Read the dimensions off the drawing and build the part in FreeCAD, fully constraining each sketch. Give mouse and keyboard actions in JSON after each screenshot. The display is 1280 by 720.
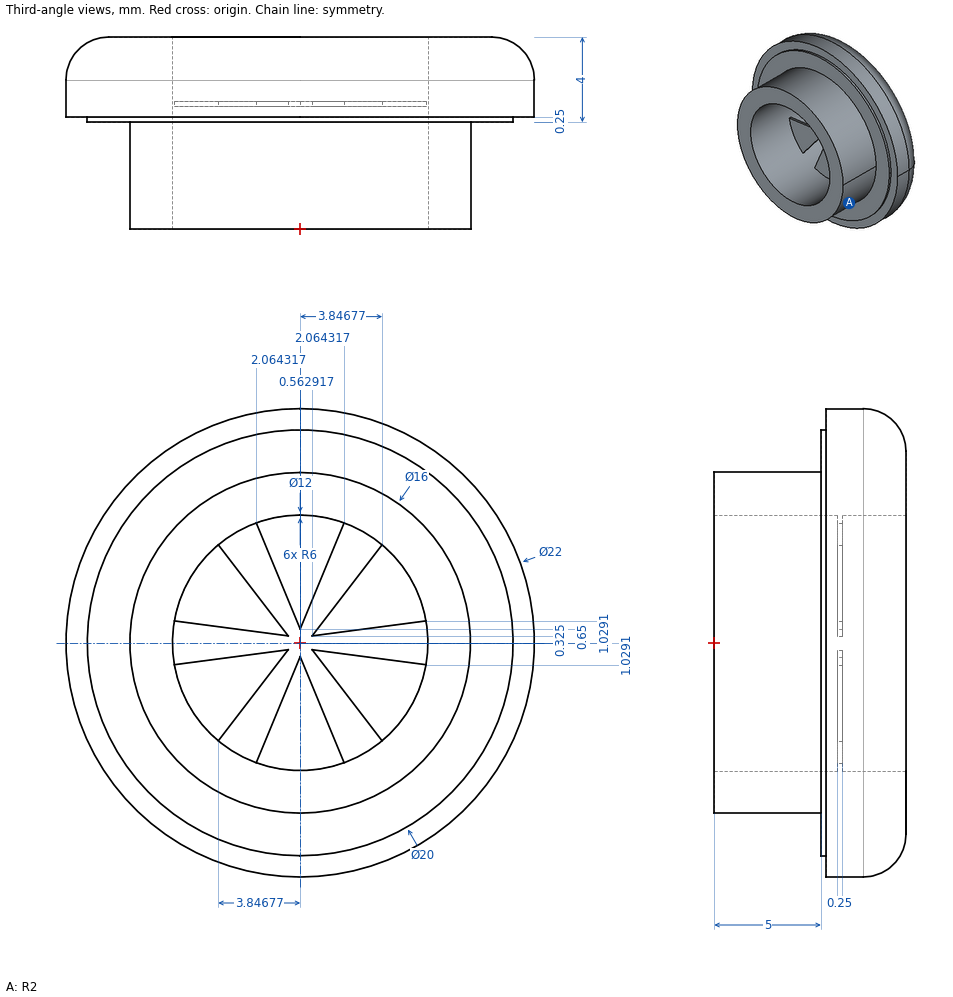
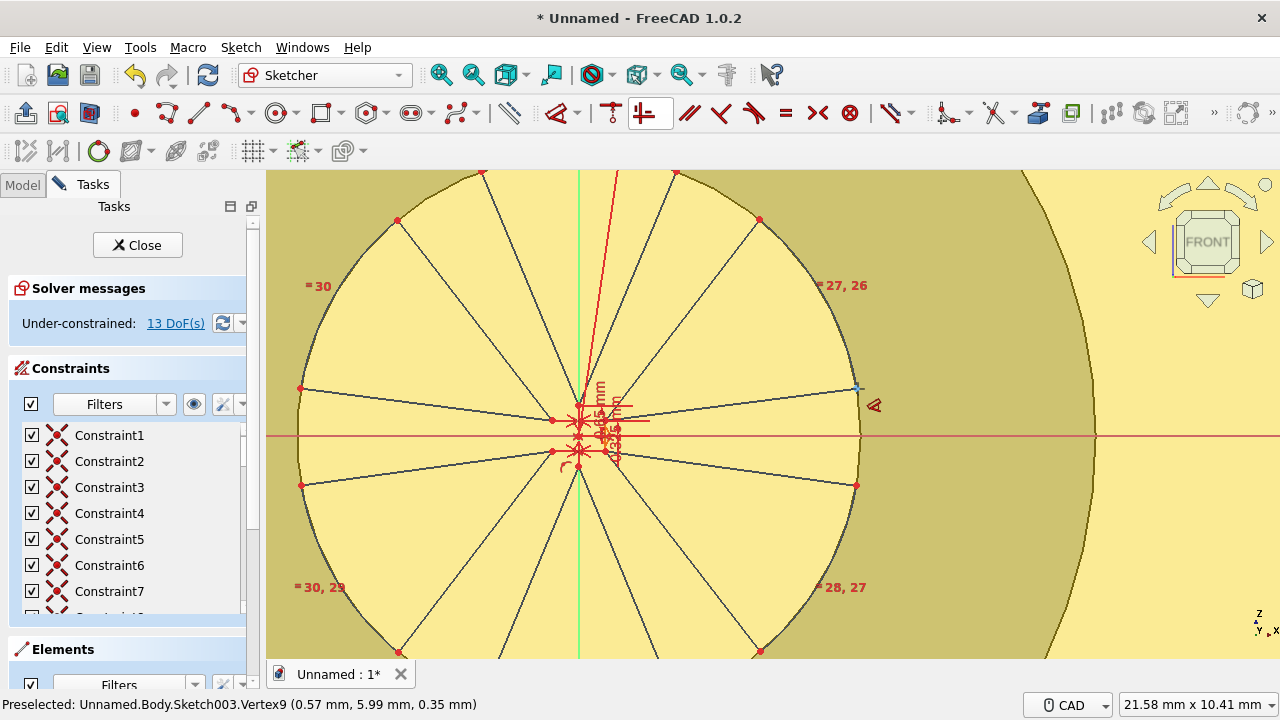
{"action": "left_click", "coordinate": [857, 389]}
{"action": "left_click", "coordinate": [891, 412]}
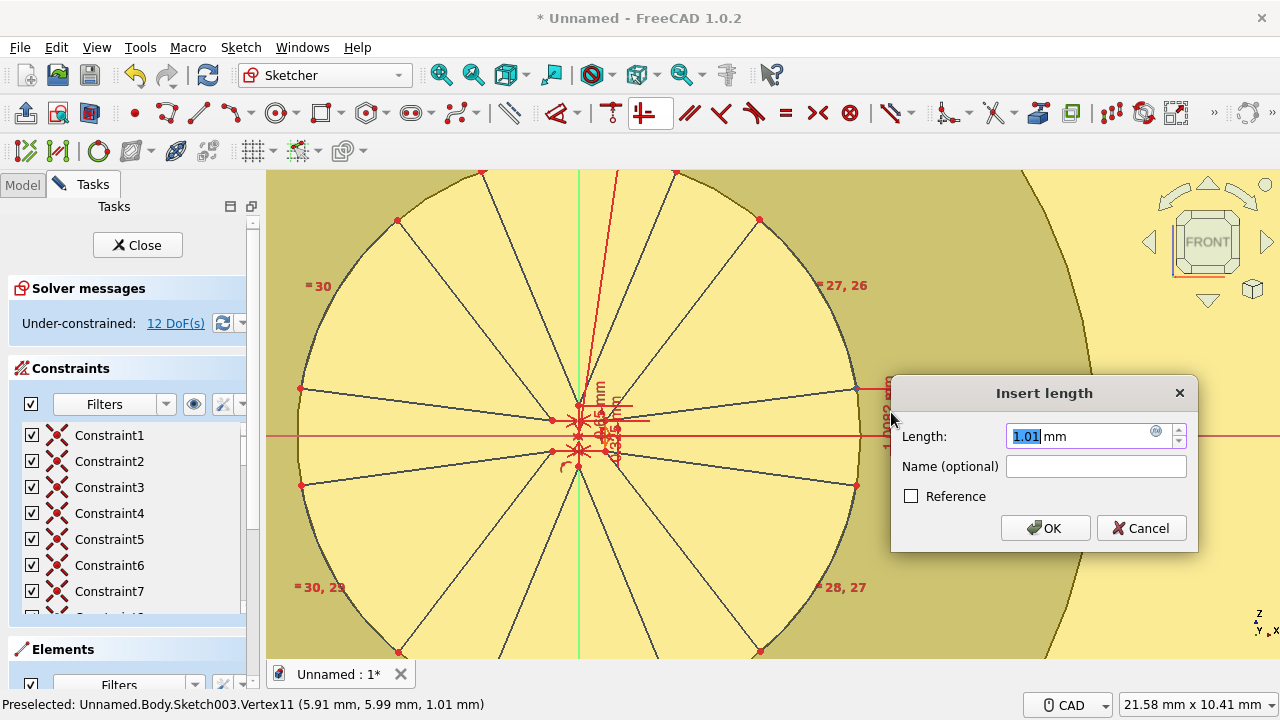
{"action": "type", "text": "1.0291"}
{"action": "key", "text": "Return"}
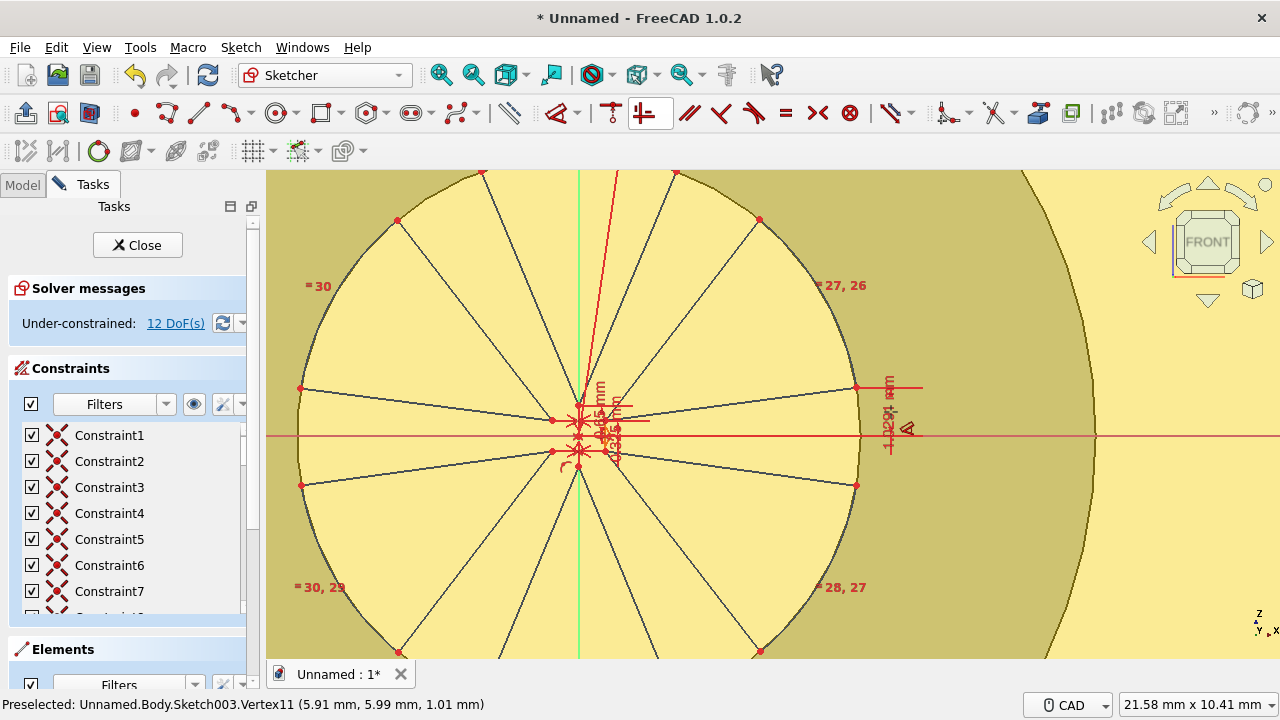
{"action": "left_click", "coordinate": [856, 486]}
{"action": "left_click", "coordinate": [890, 461]}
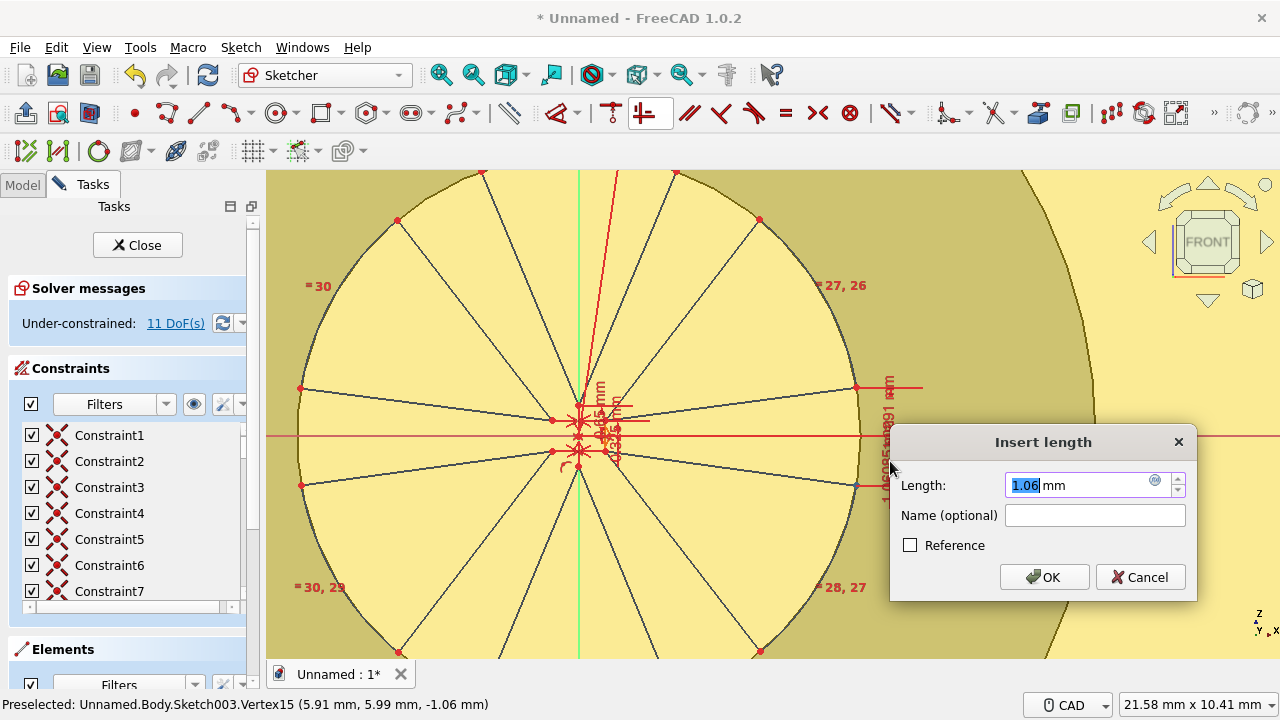
{"action": "type", "text": "1.0291"}
{"action": "key", "text": "Return"}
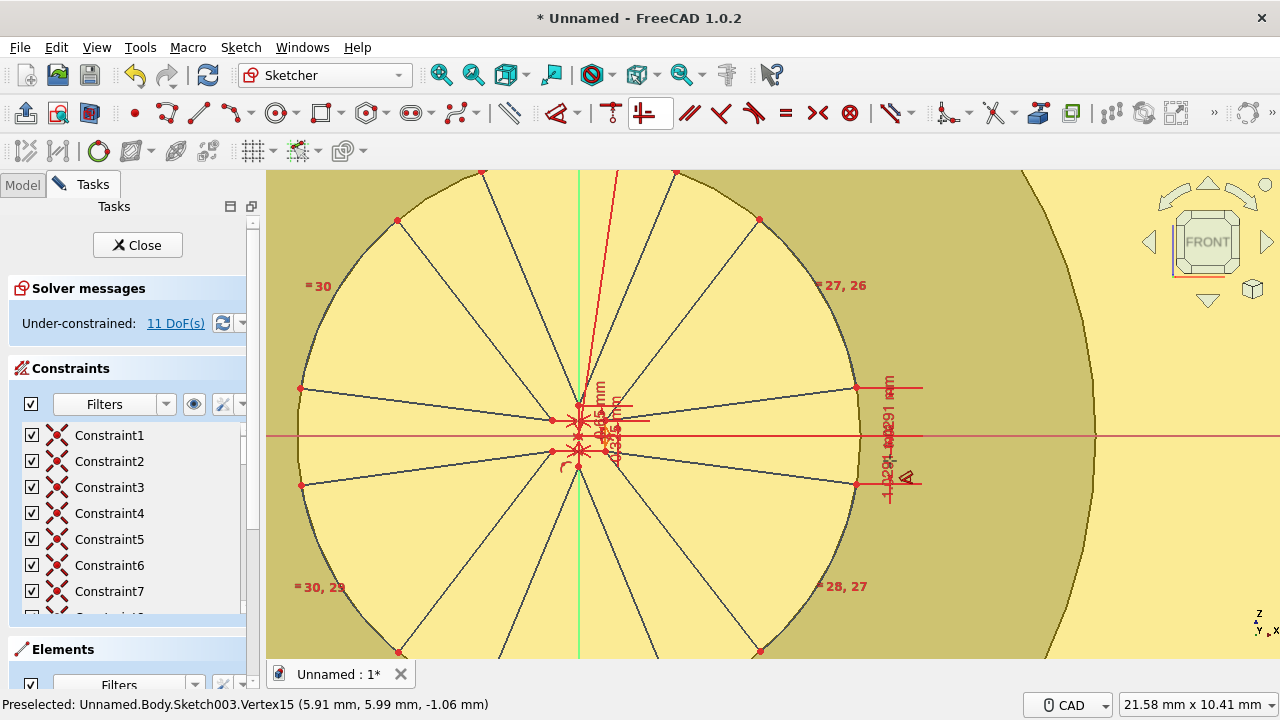
{"action": "left_click", "coordinate": [301, 486]}
{"action": "left_click", "coordinate": [661, 472]}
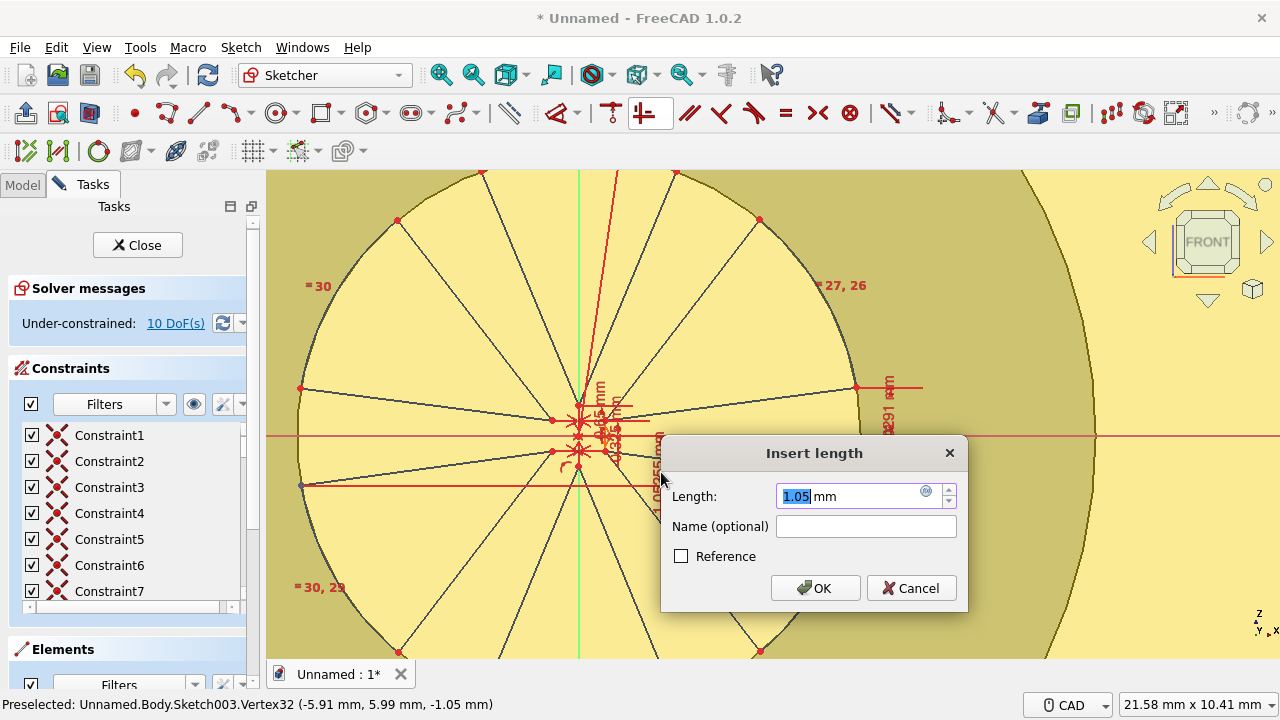
{"action": "type", "text": "1.0291"}
{"action": "key", "text": "Return"}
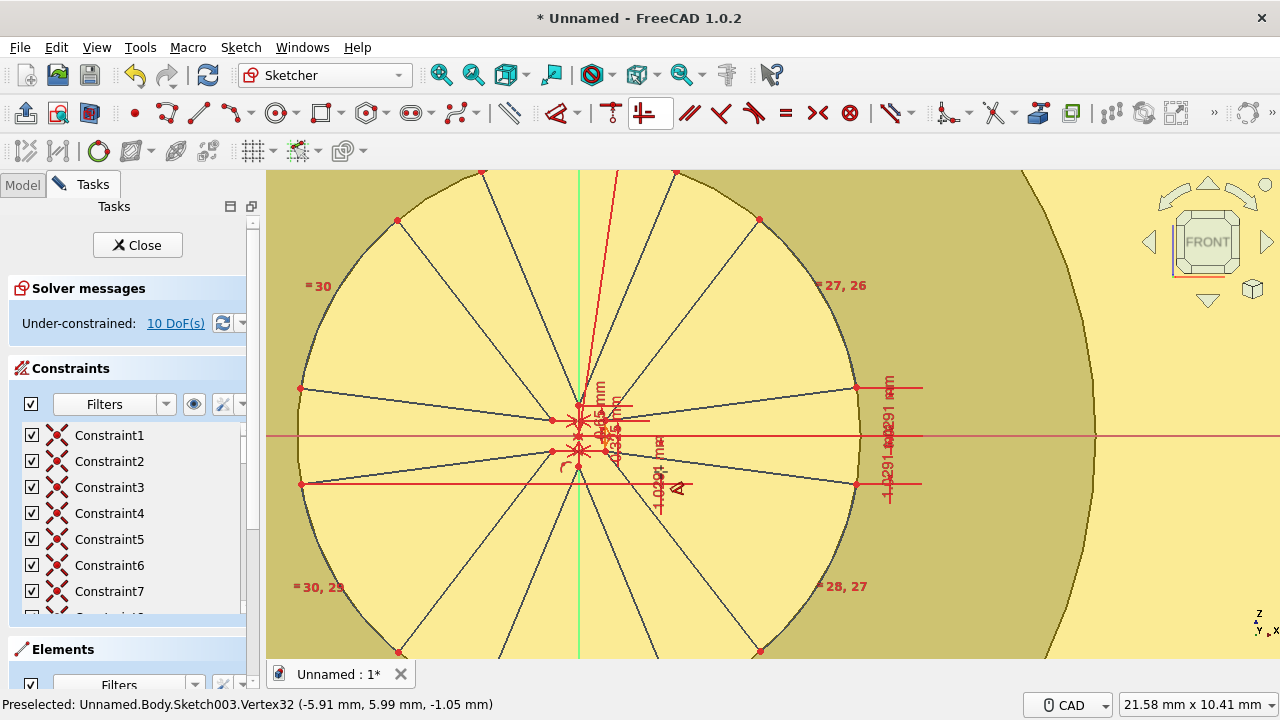
{"action": "left_click", "coordinate": [301, 389]}
{"action": "left_click", "coordinate": [685, 396]}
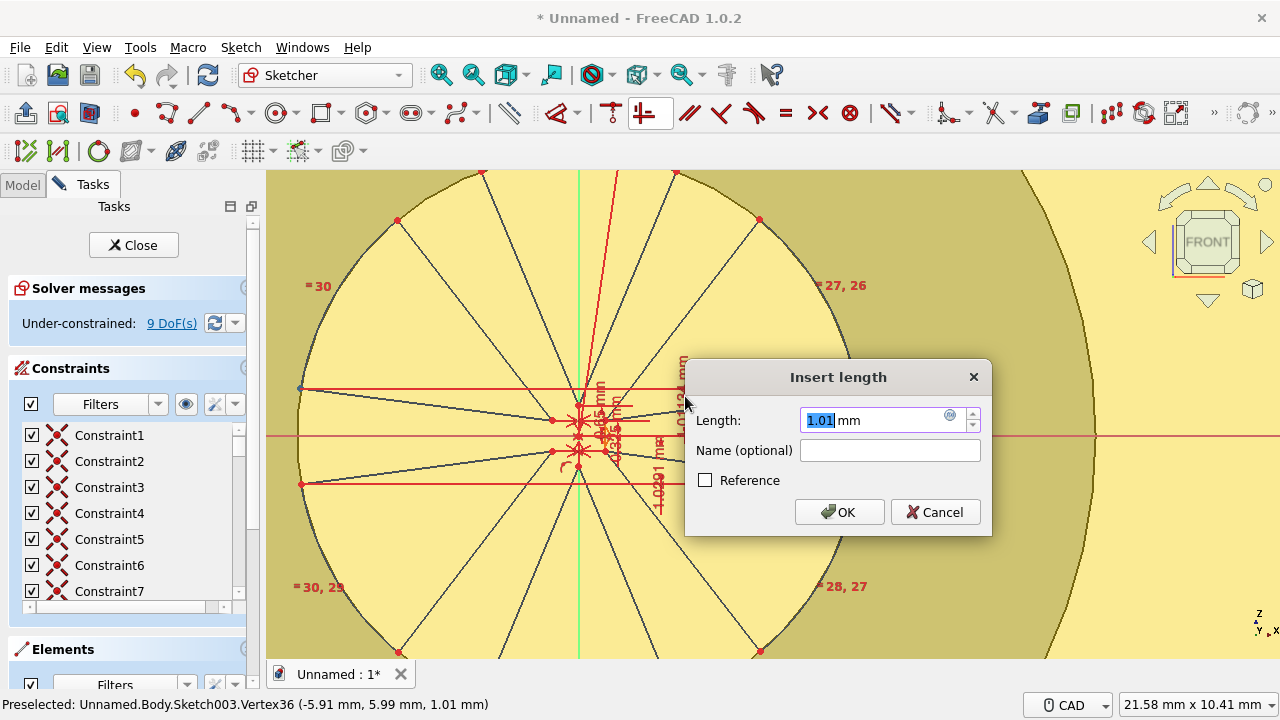
{"action": "type", "text": "1.0291"}
{"action": "key", "text": "Return"}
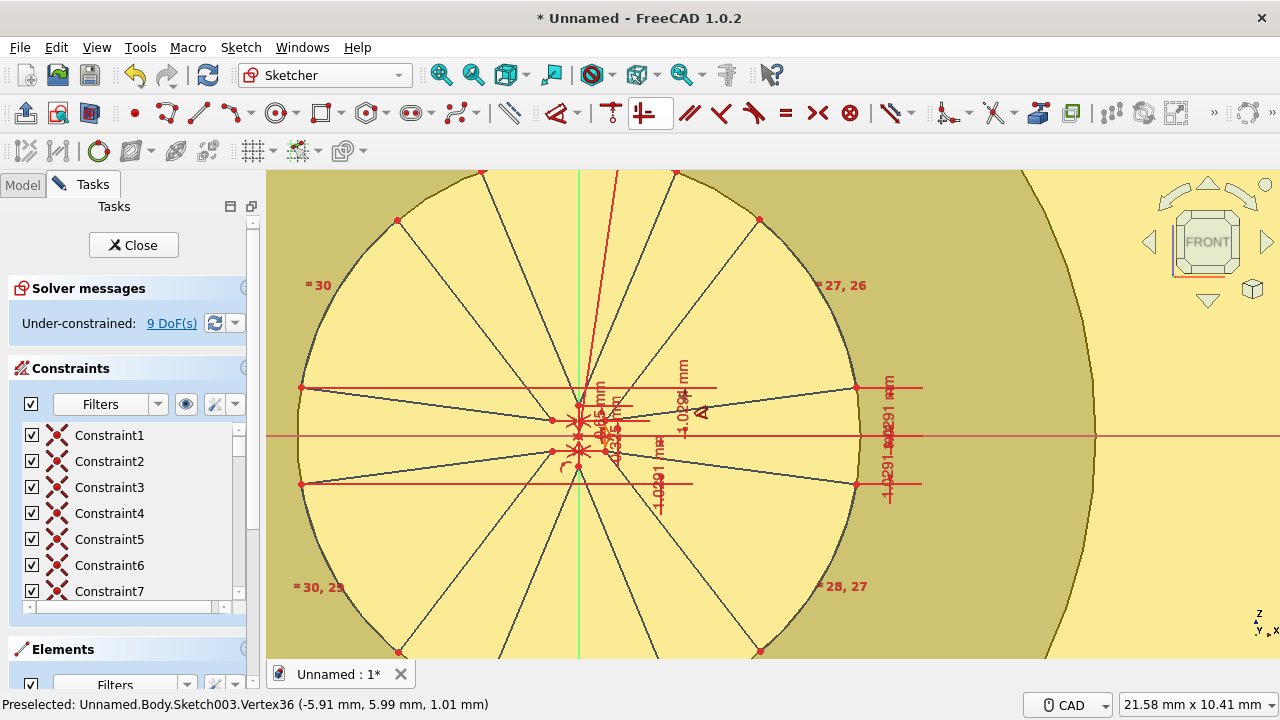
{"action": "left_click", "coordinate": [760, 220]}
{"action": "left_click", "coordinate": [669, 494]}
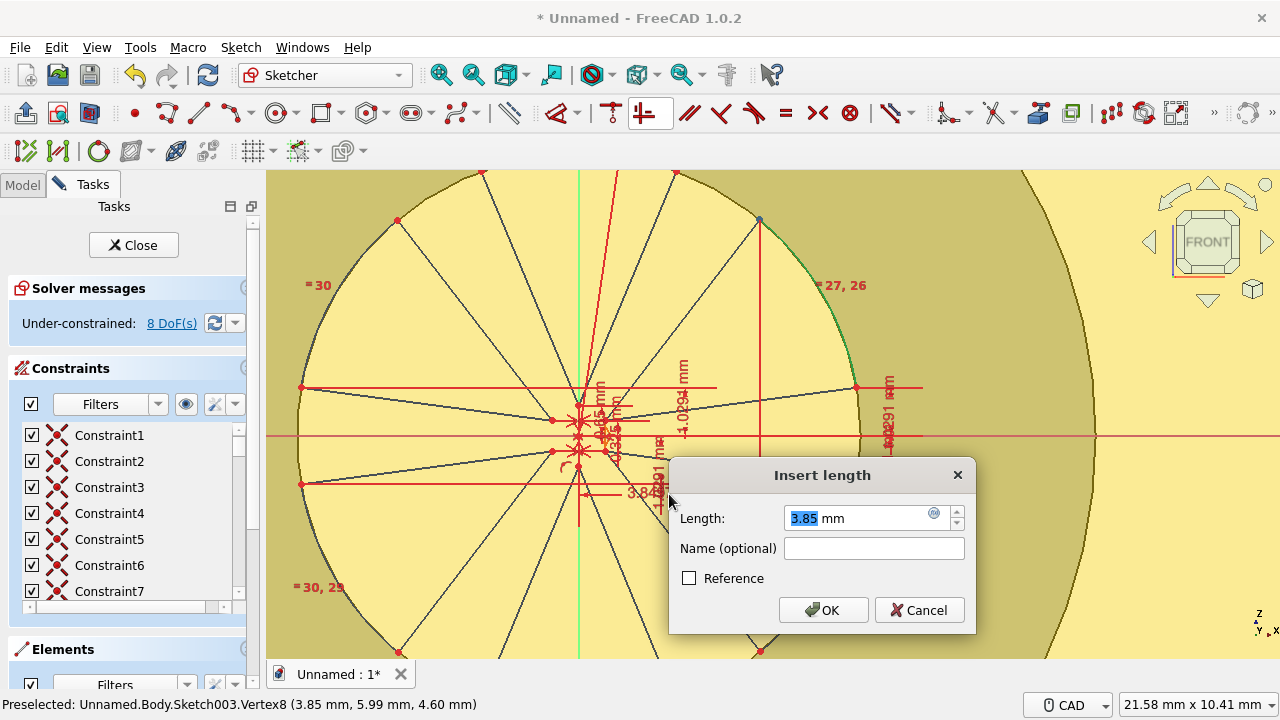
{"action": "type", "text": "3.84677"}
{"action": "key", "text": "Return"}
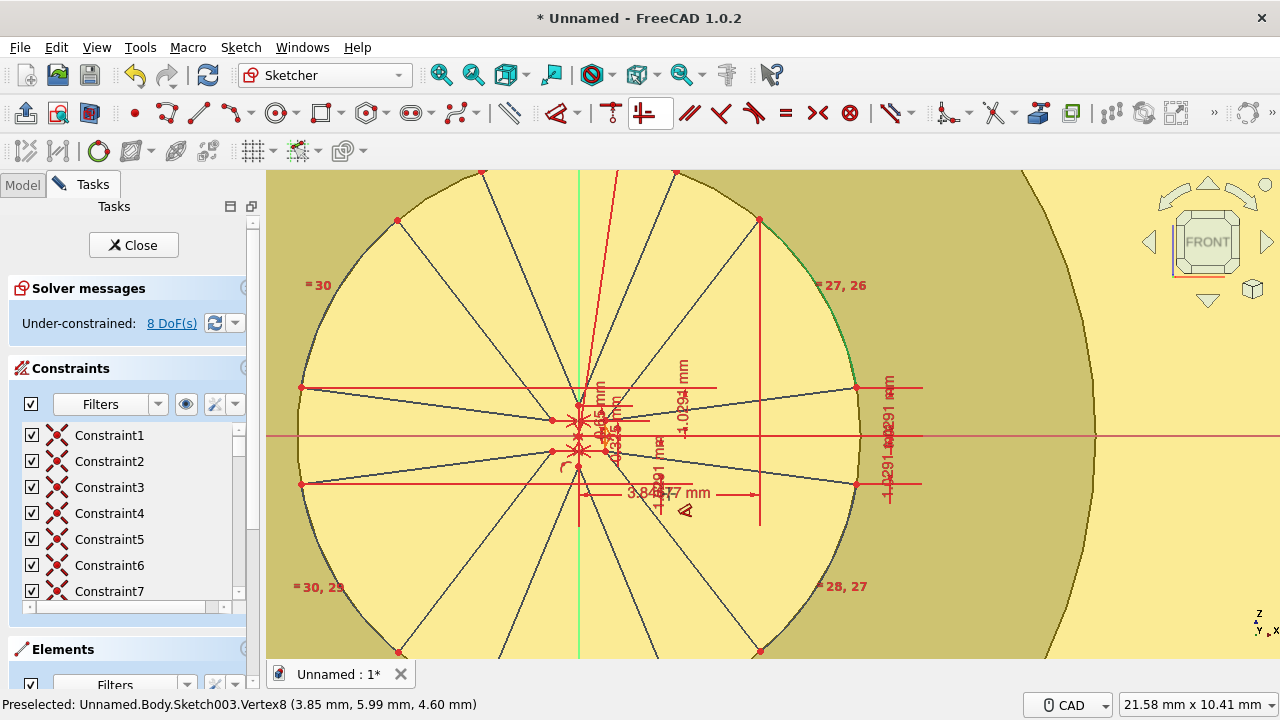
{"action": "scroll", "coordinate": [857, 388], "scroll_direction": "down", "scroll_amount": 3}